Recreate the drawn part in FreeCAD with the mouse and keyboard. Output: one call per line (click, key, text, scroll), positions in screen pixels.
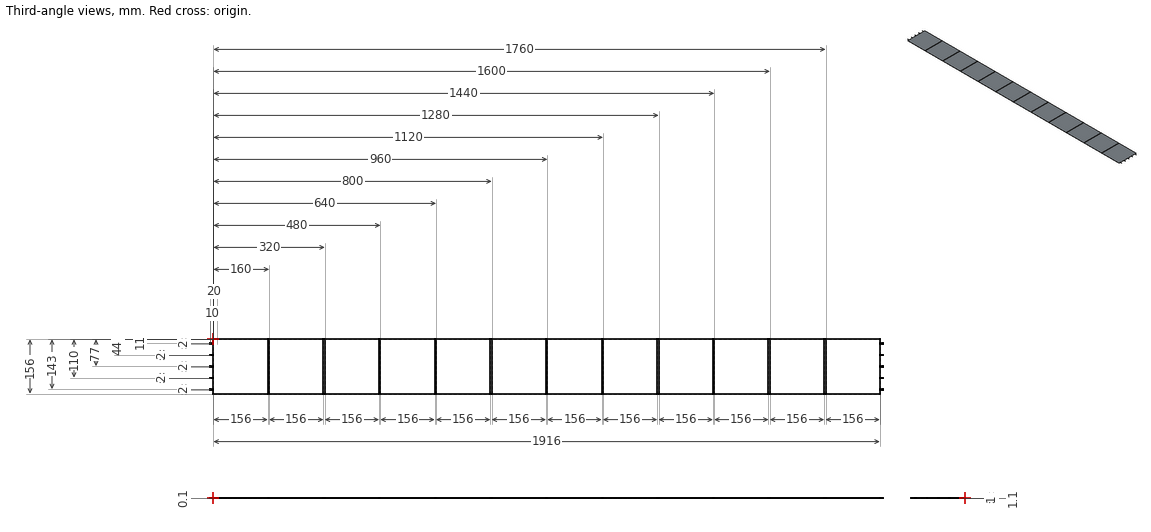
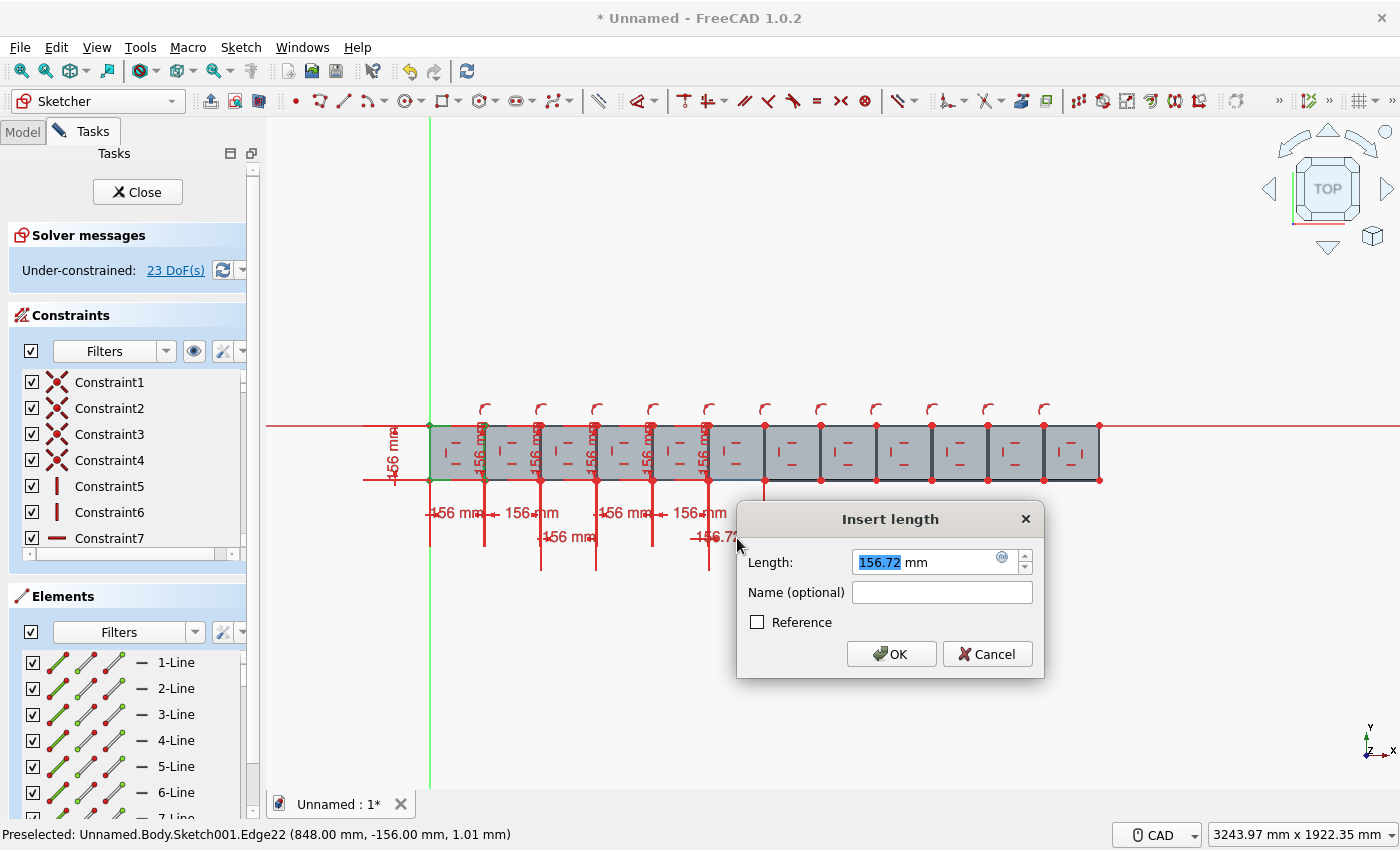
text(156)
key(Return)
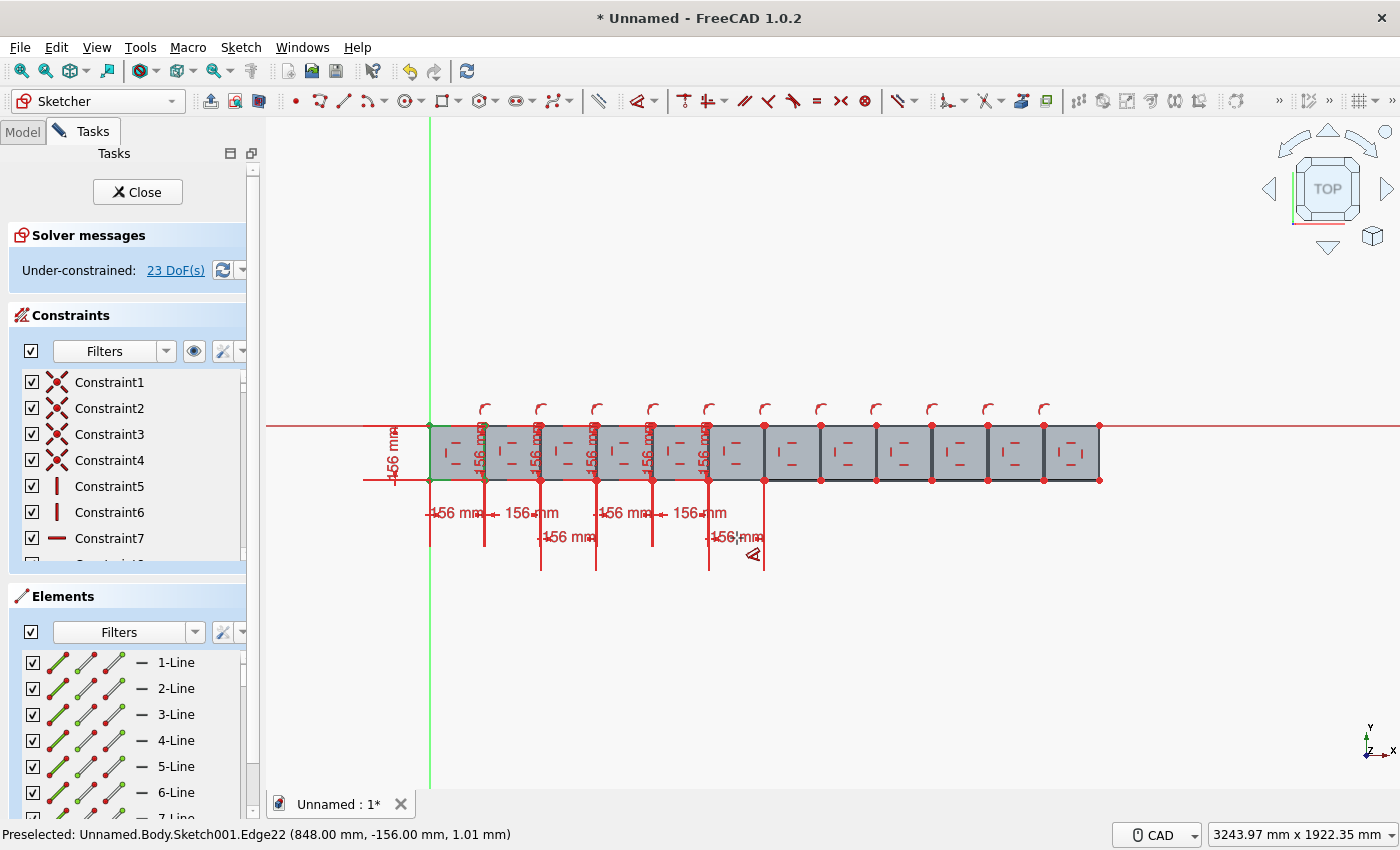
scroll(765, 442, up, 12)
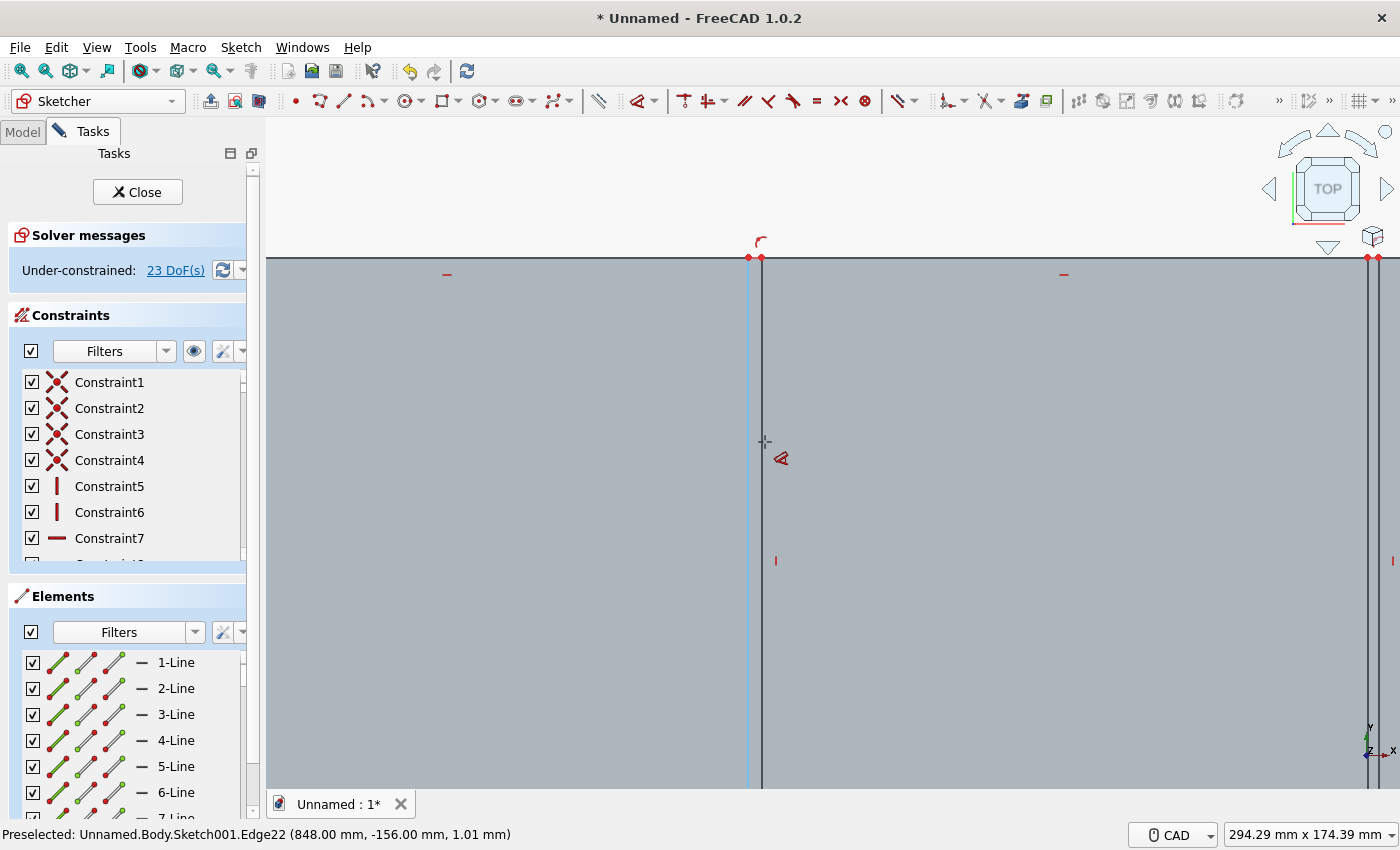
click(762, 441)
click(796, 509)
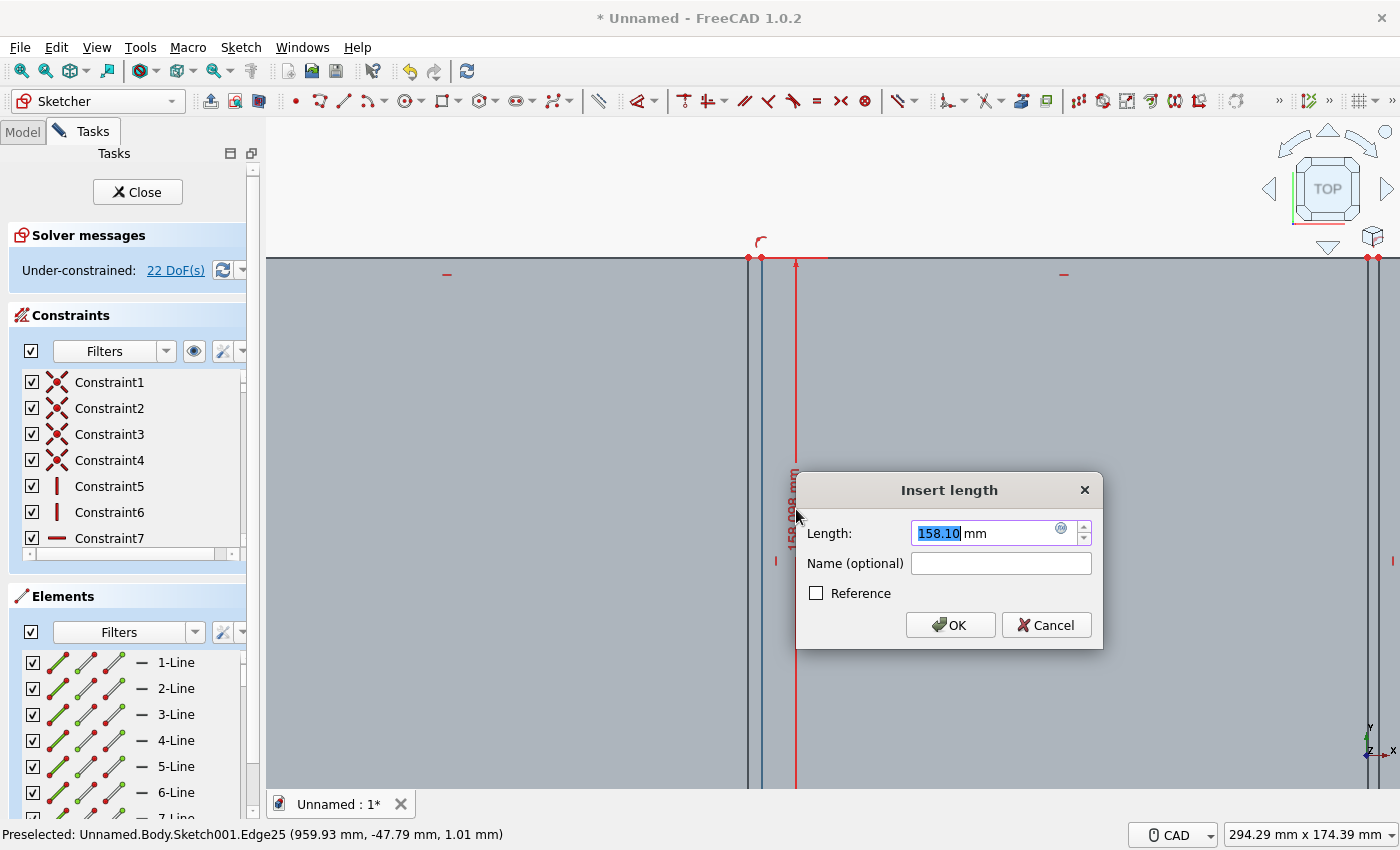
text(156)
key(Return)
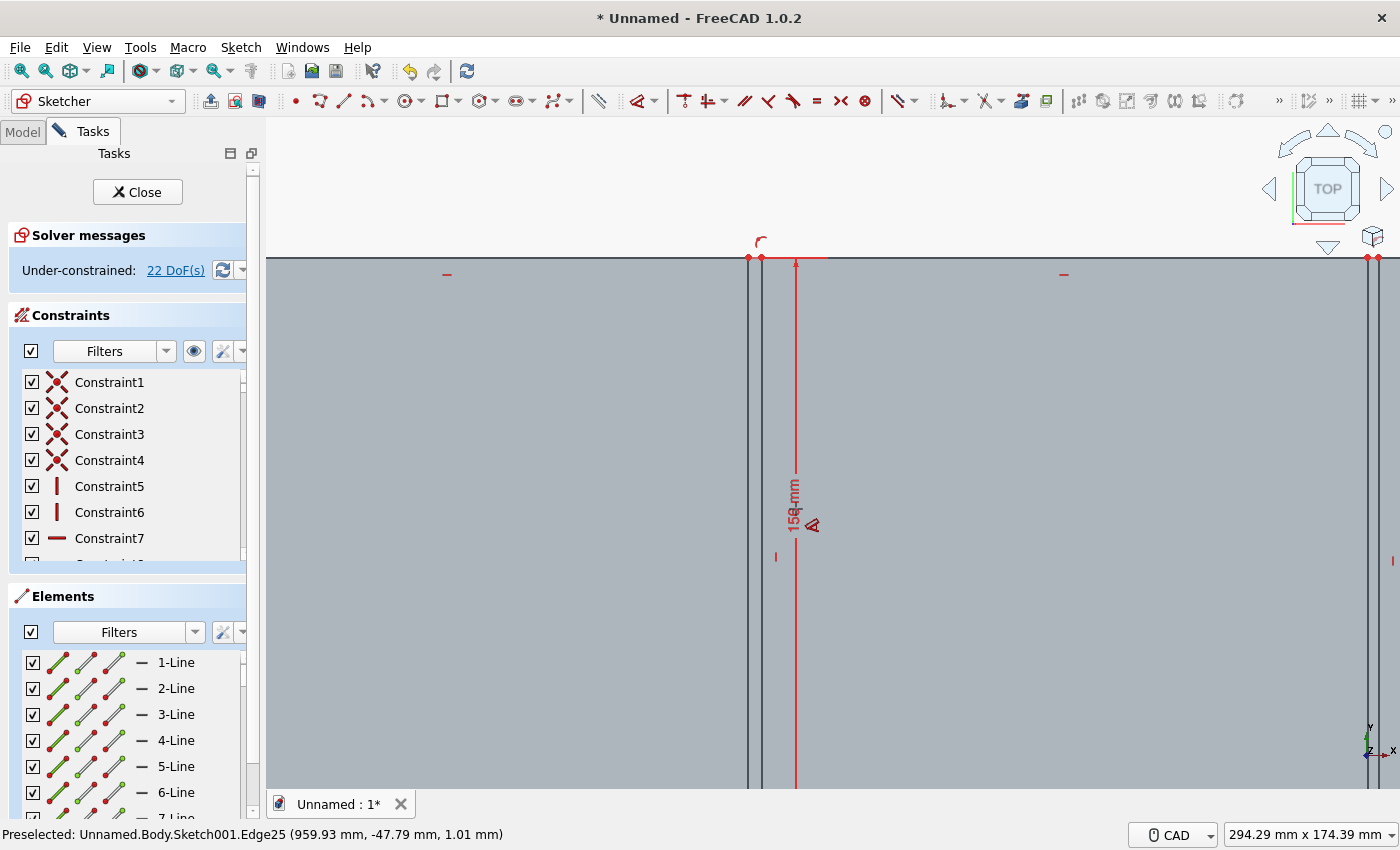
scroll(765, 442, down, 12)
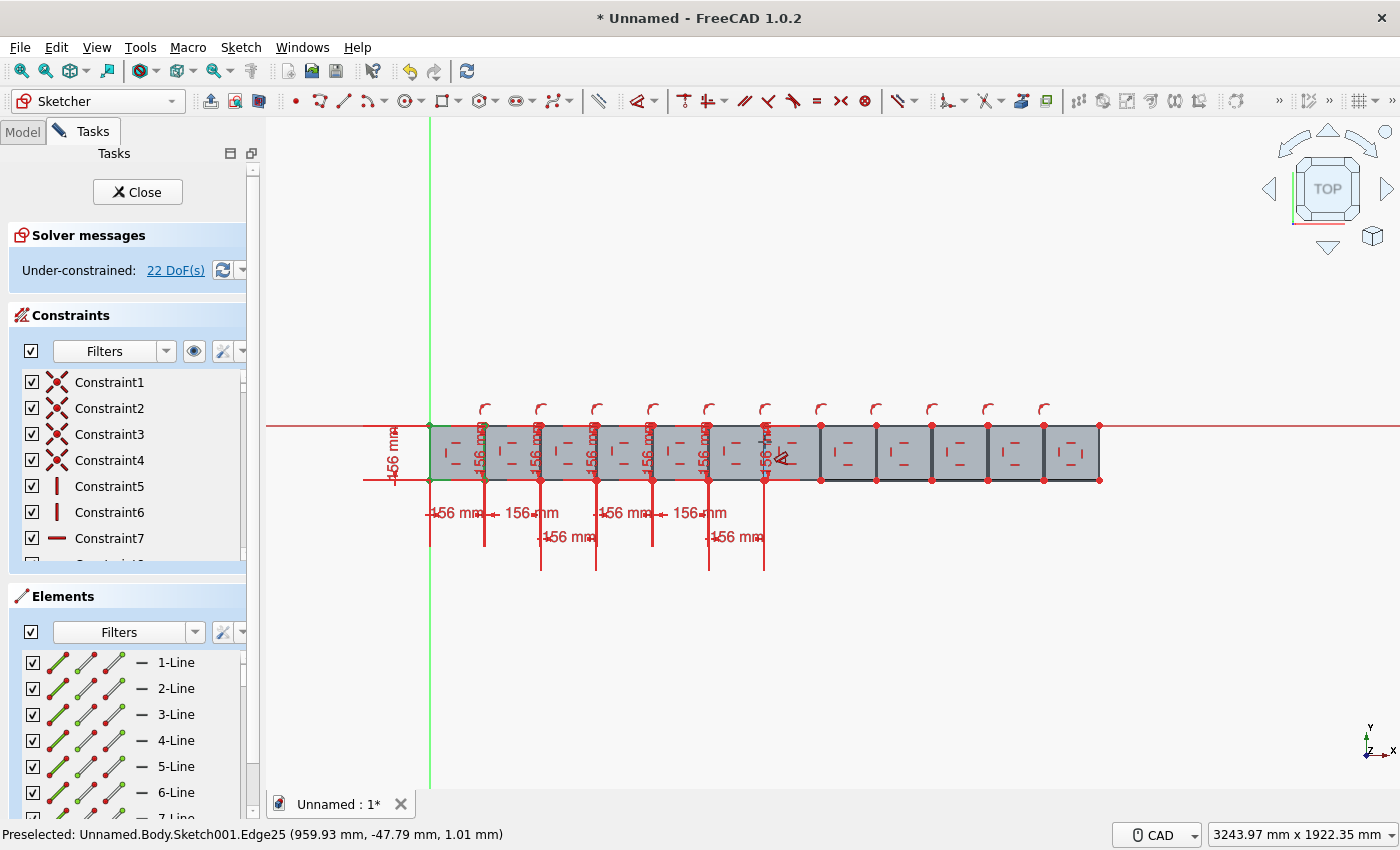
click(782, 480)
click(793, 514)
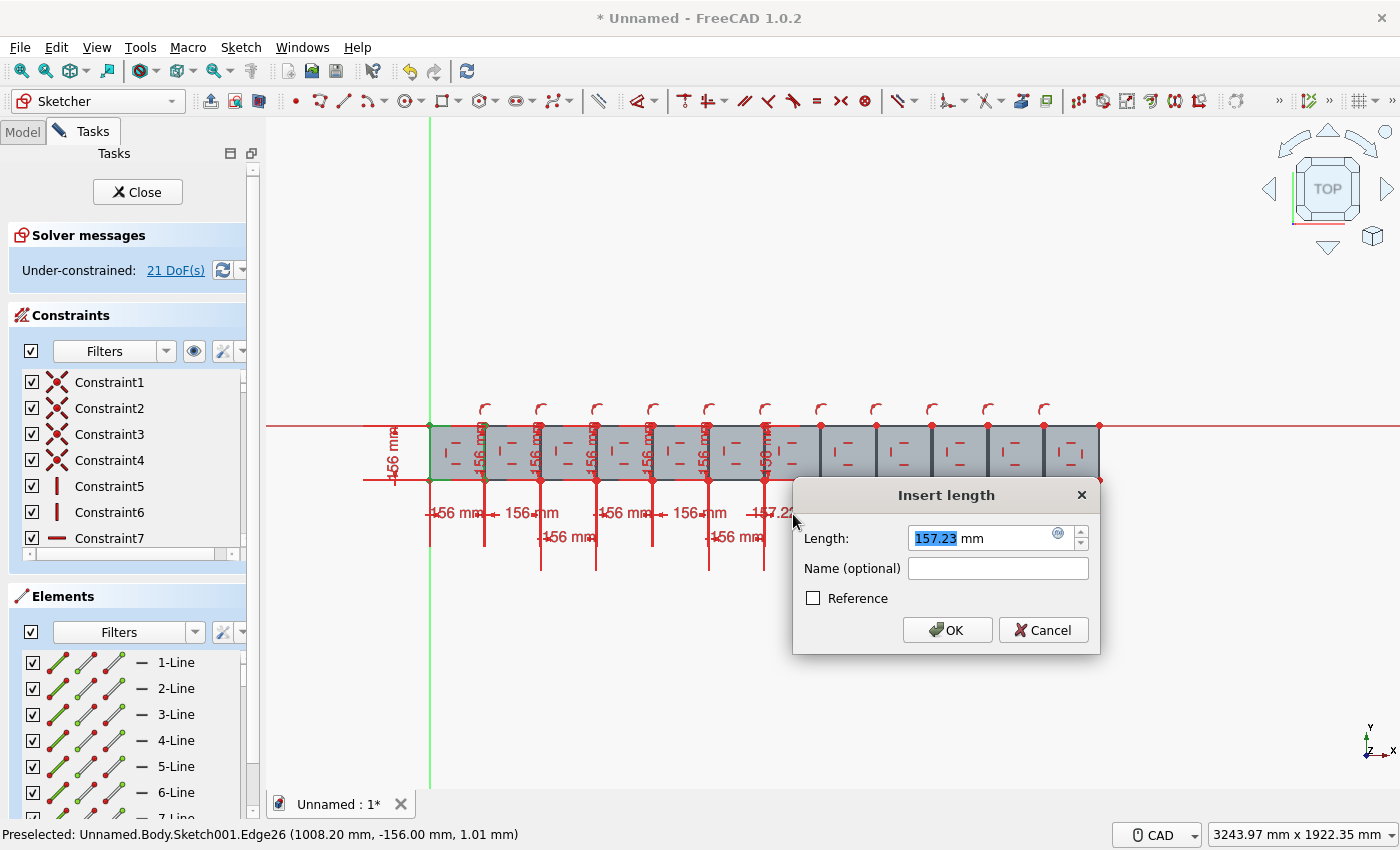
text(156)
key(Return)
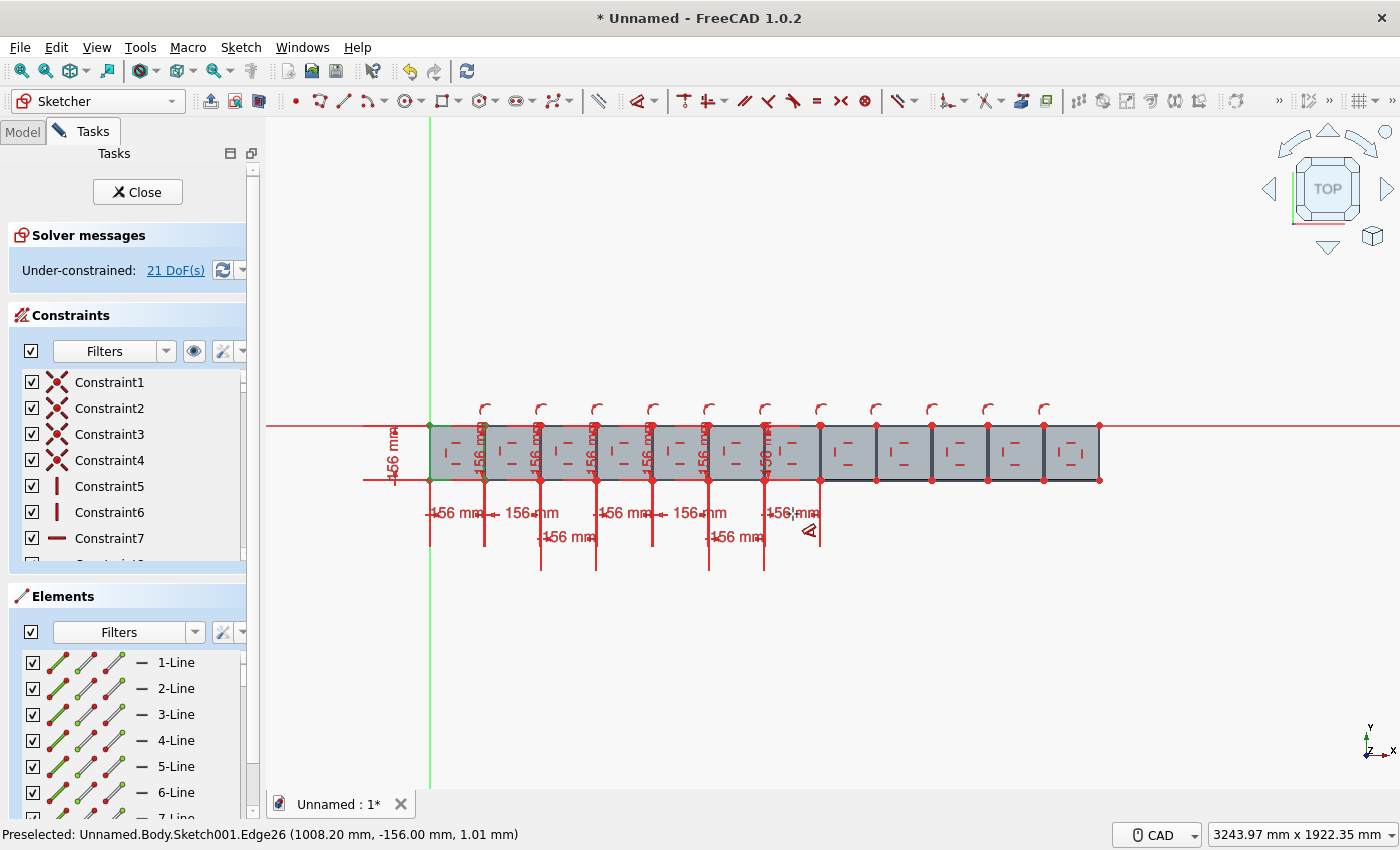
scroll(821, 442, up, 12)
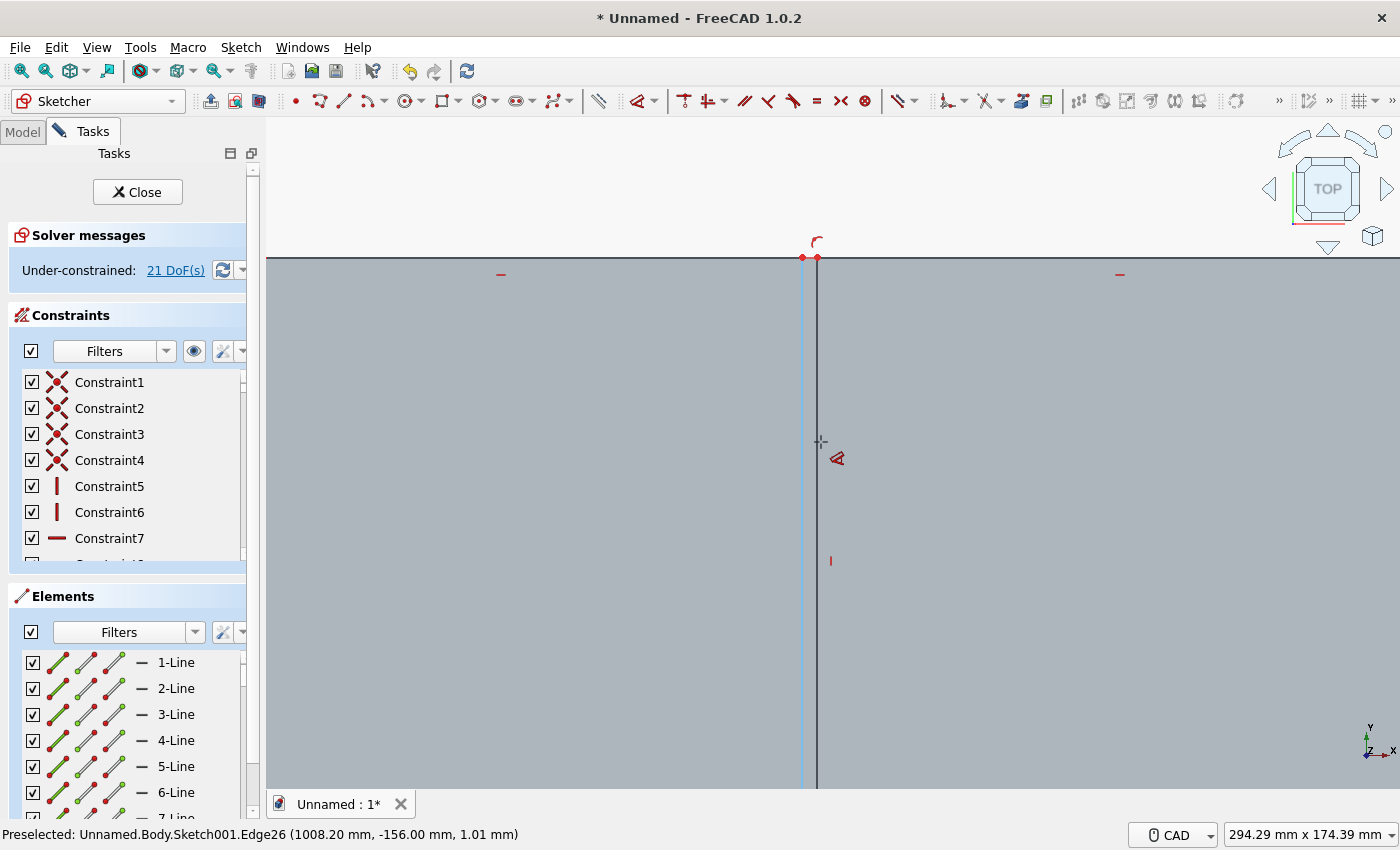
click(817, 441)
click(851, 509)